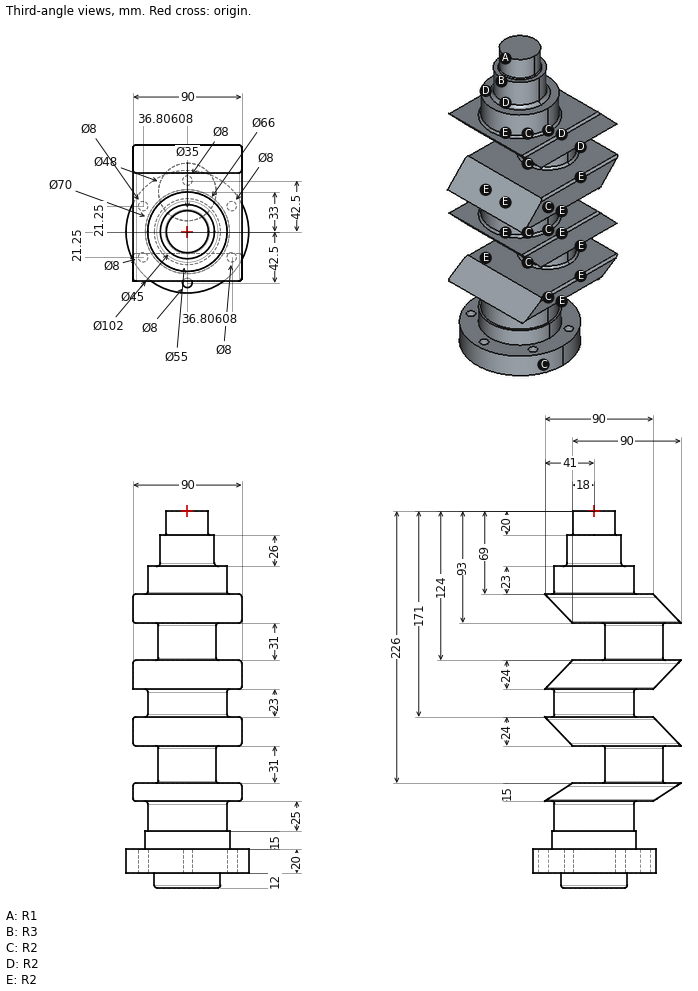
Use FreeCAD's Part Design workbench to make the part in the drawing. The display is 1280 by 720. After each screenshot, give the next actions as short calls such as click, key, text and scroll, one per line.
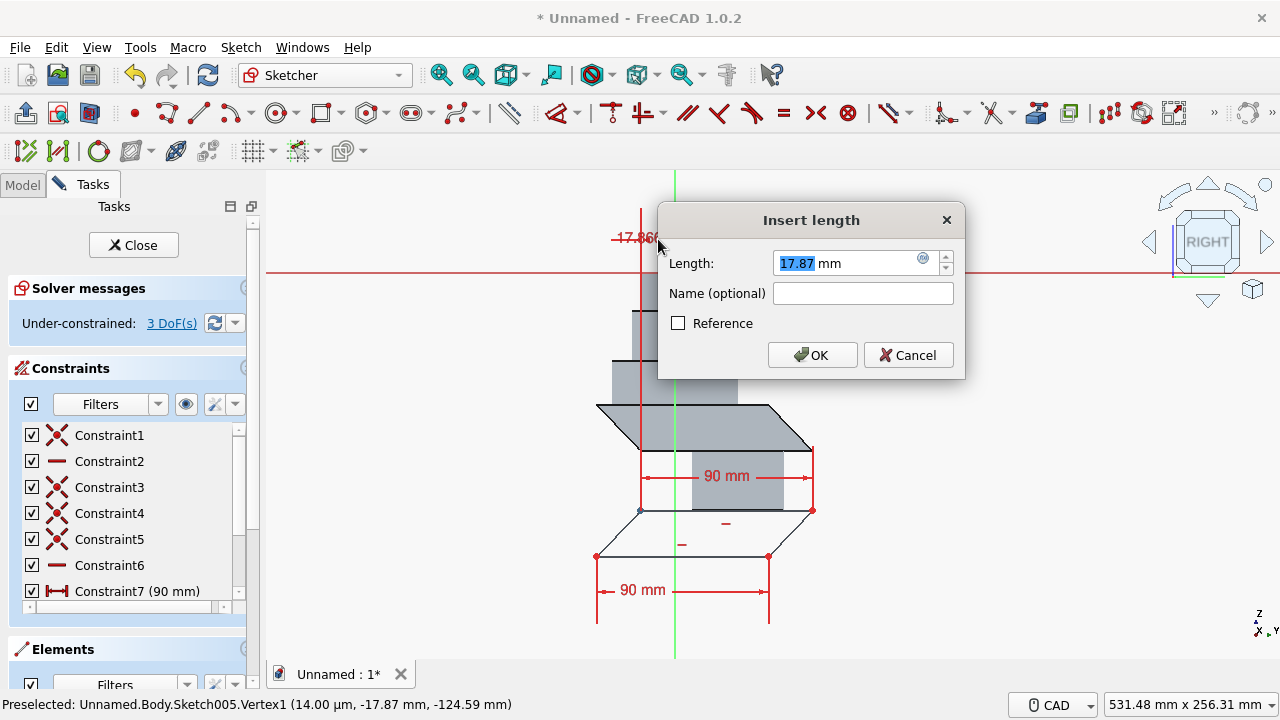
text(18)
key(Return)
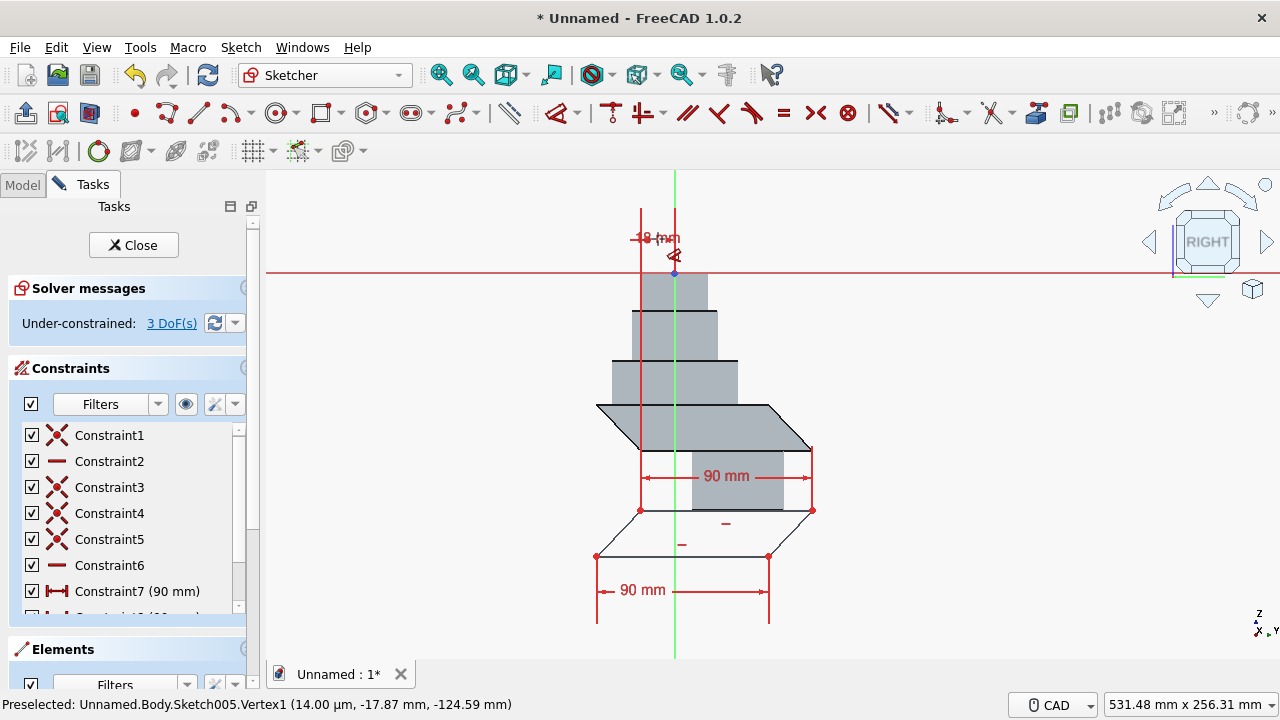
click(597, 557)
click(636, 615)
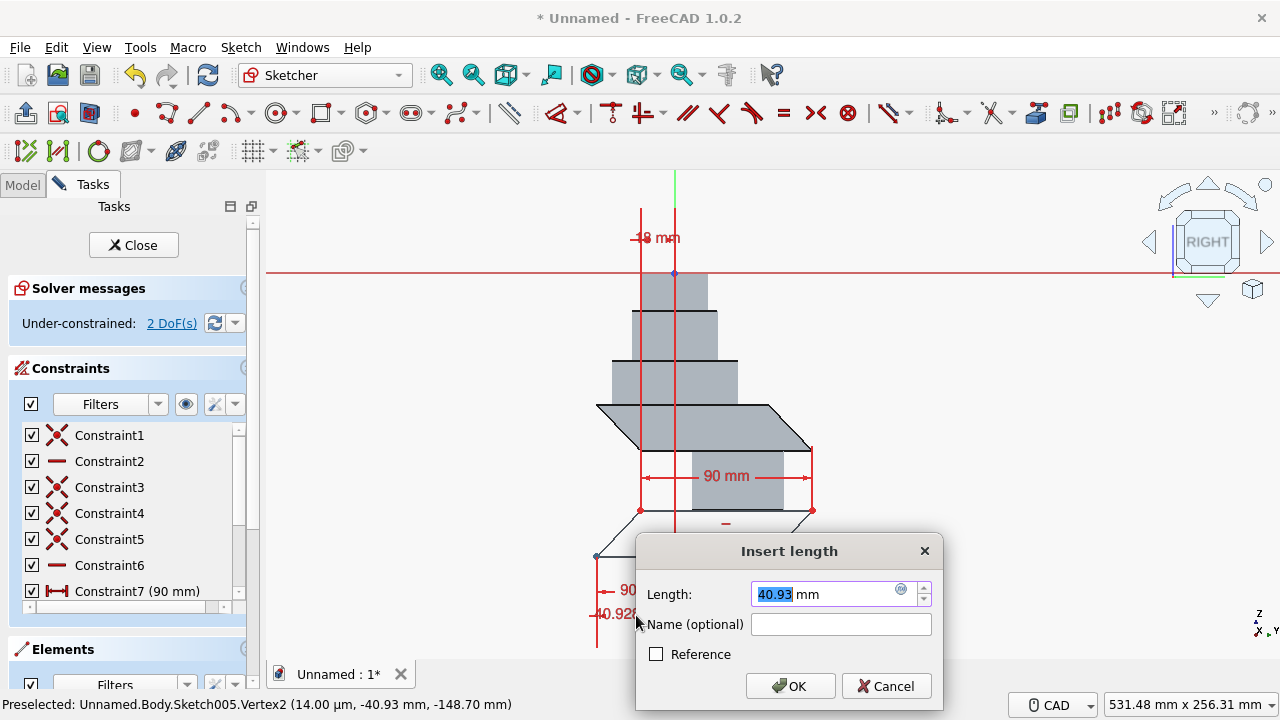
text(41)
key(Return)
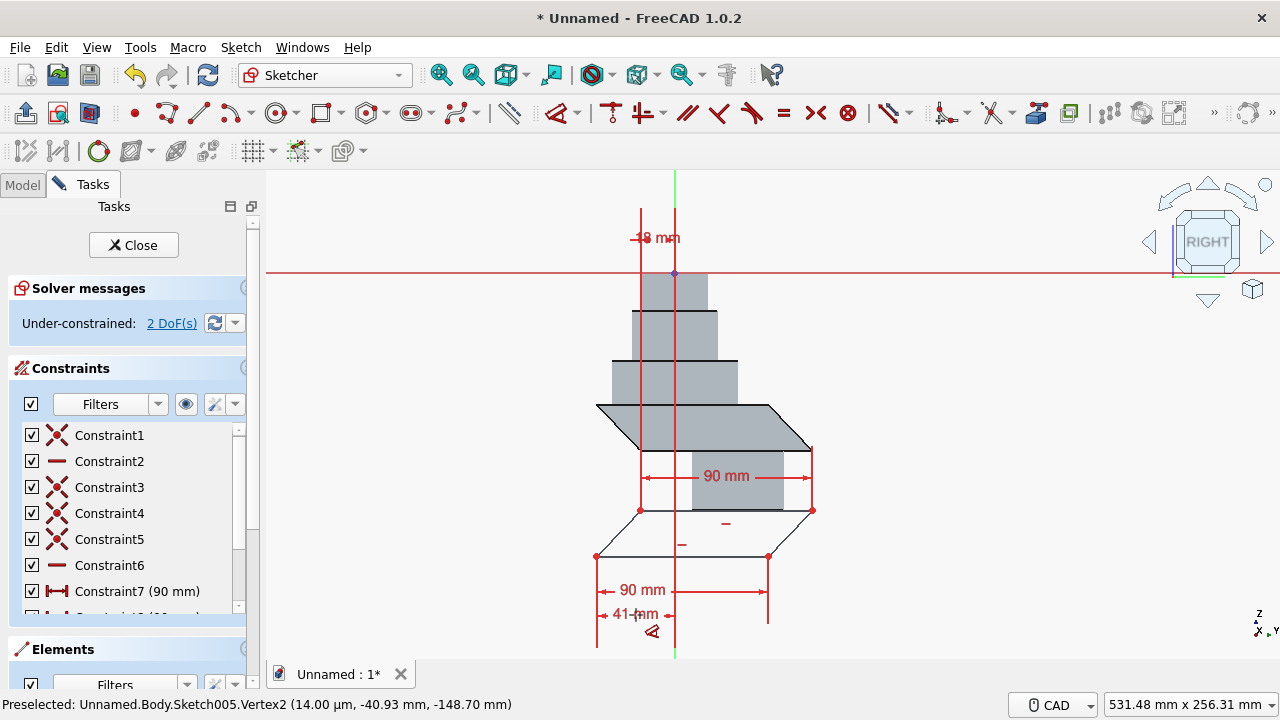
click(627, 525)
click(563, 534)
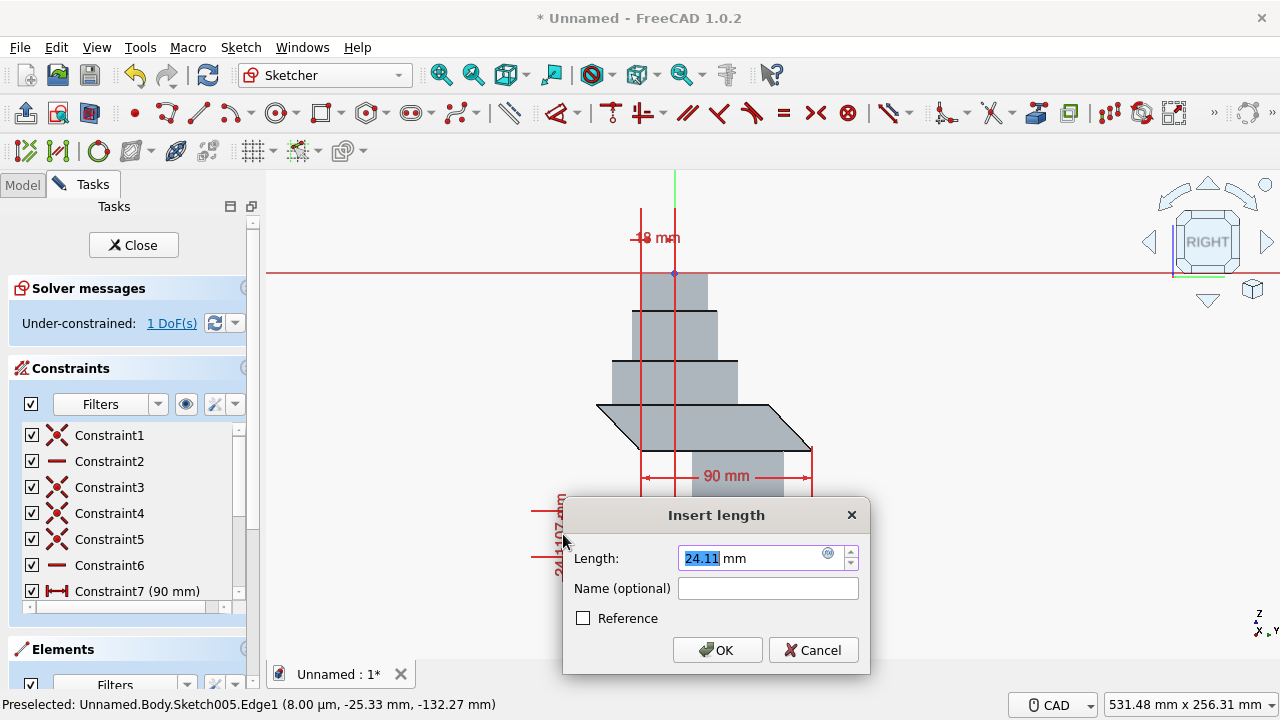
text(24)
key(Return)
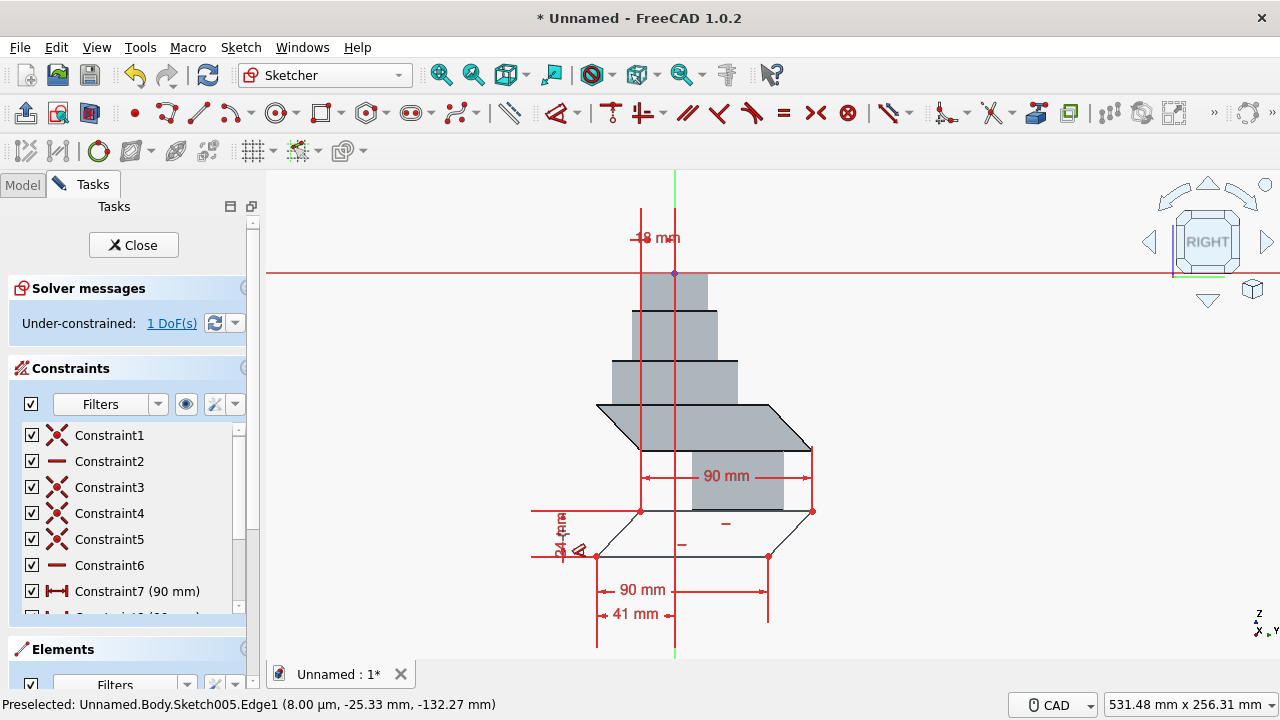
click(641, 511)
click(607, 392)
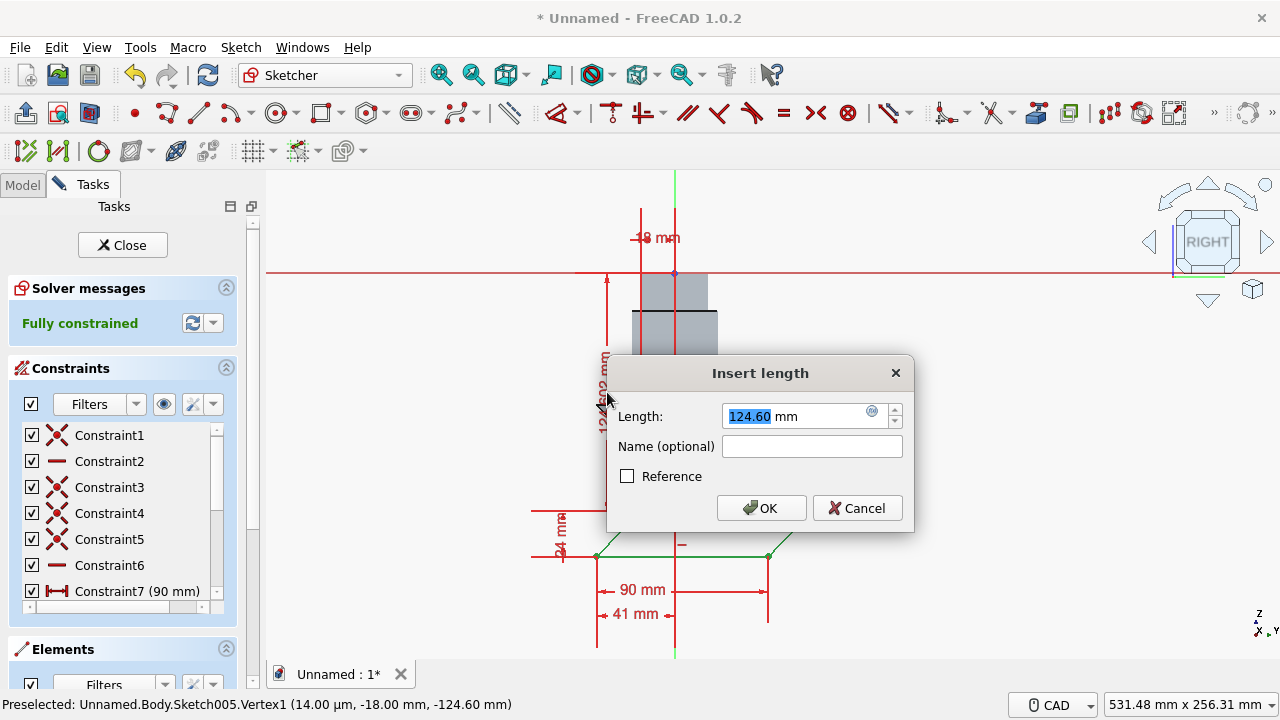
text(124)
key(Return)
key(Escape)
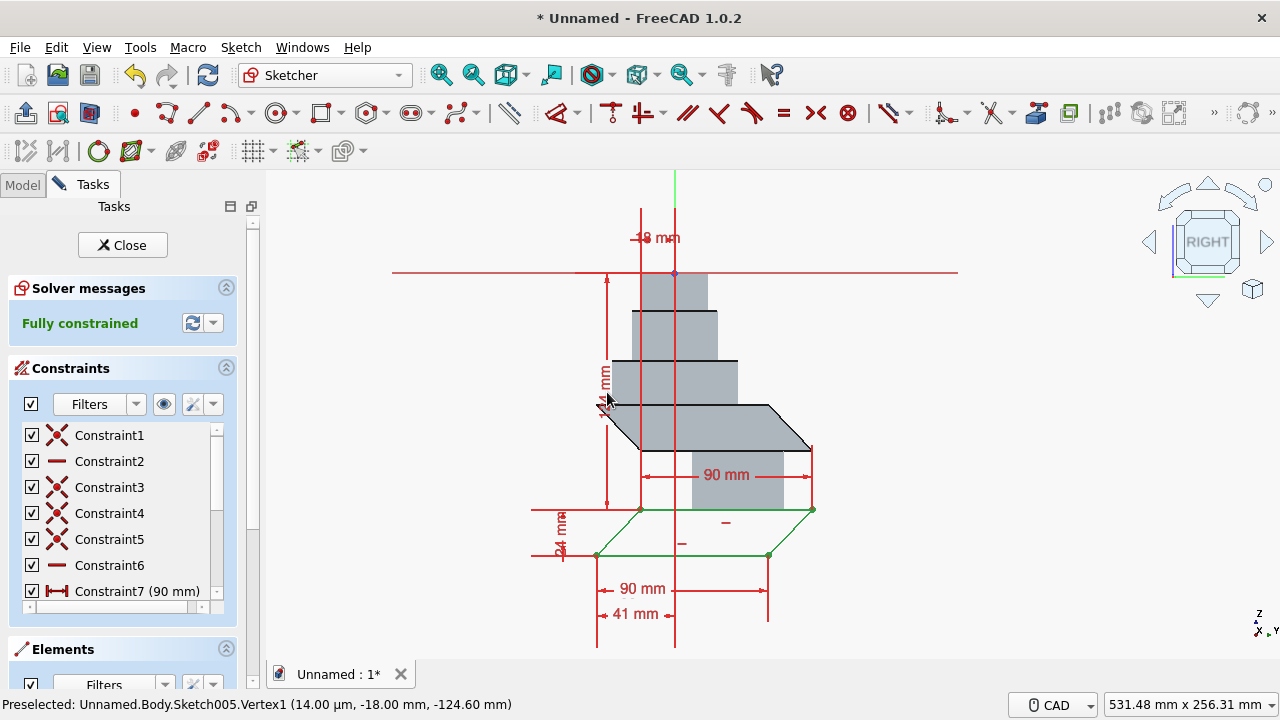
click(123, 245)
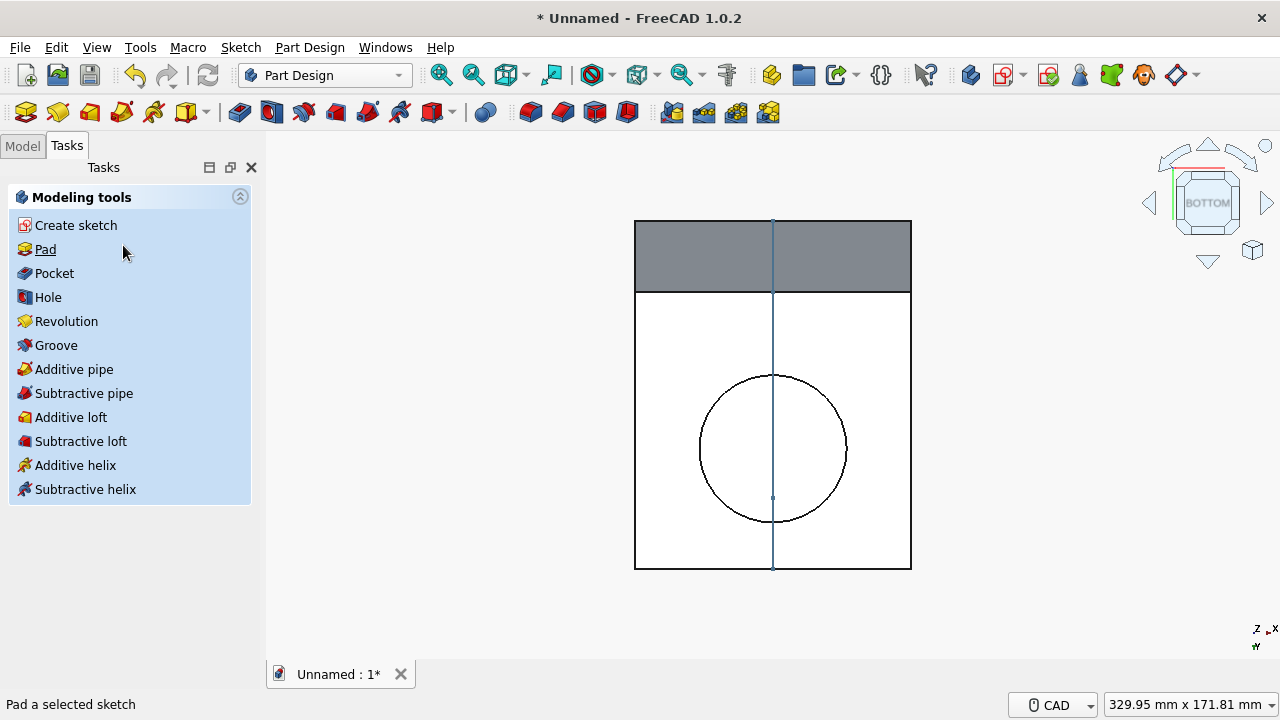
click(26, 112)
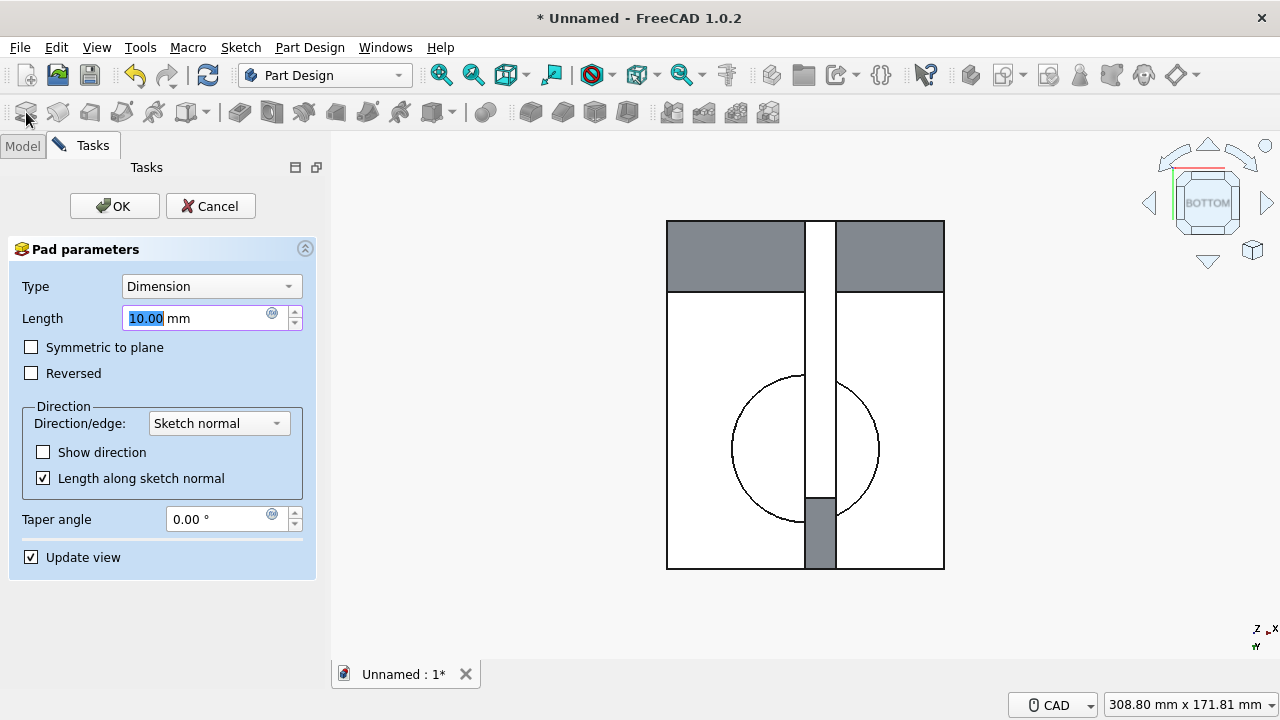
text(90)
key(Tab)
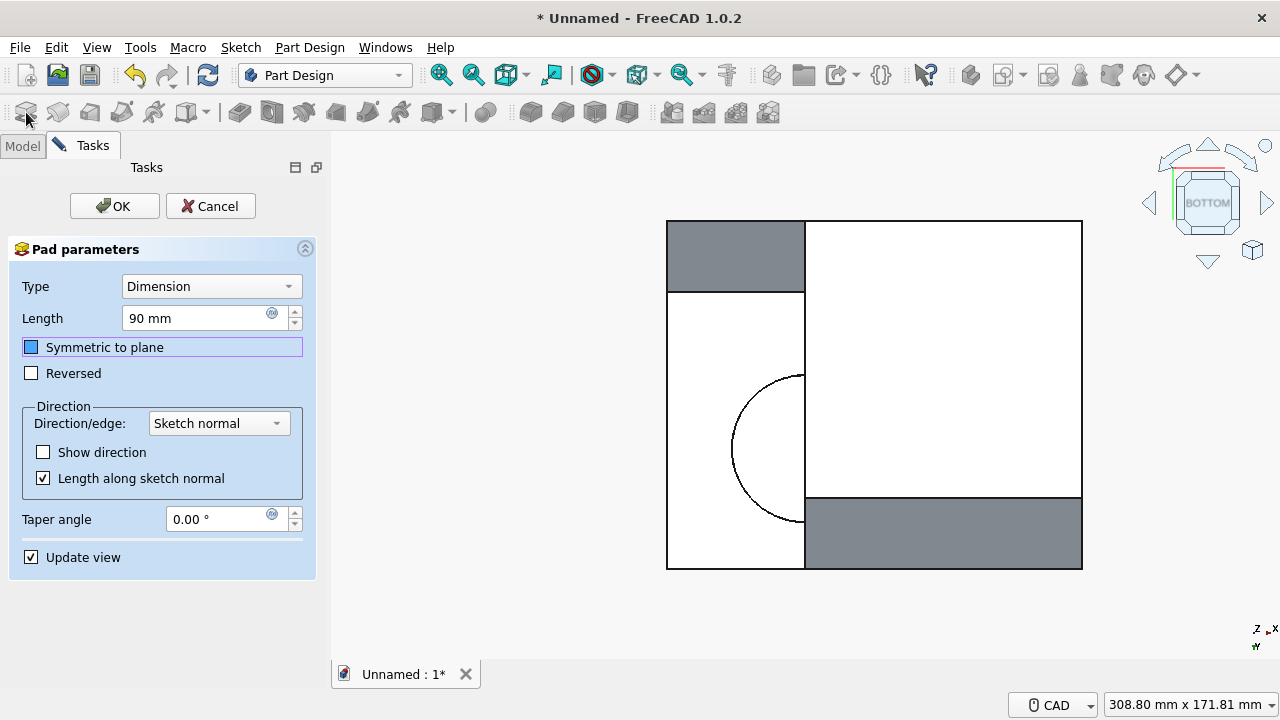
click(30, 347)